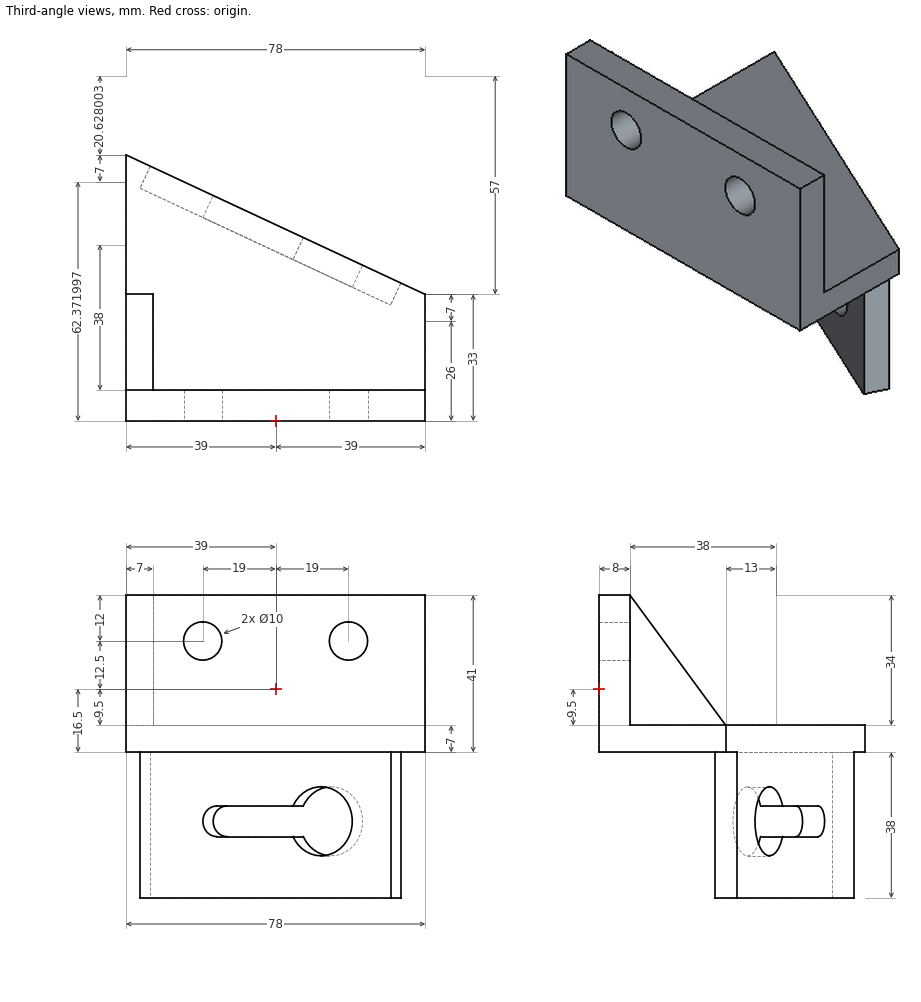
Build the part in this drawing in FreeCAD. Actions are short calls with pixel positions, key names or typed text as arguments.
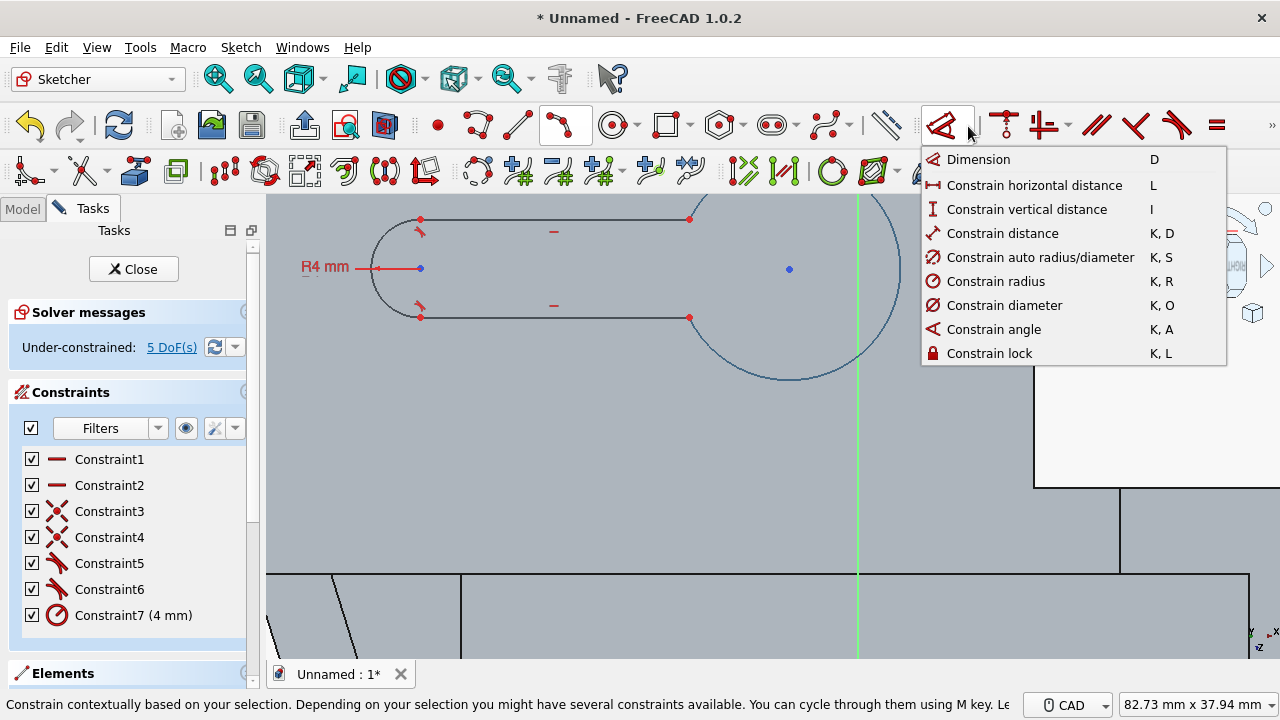
click(1074, 281)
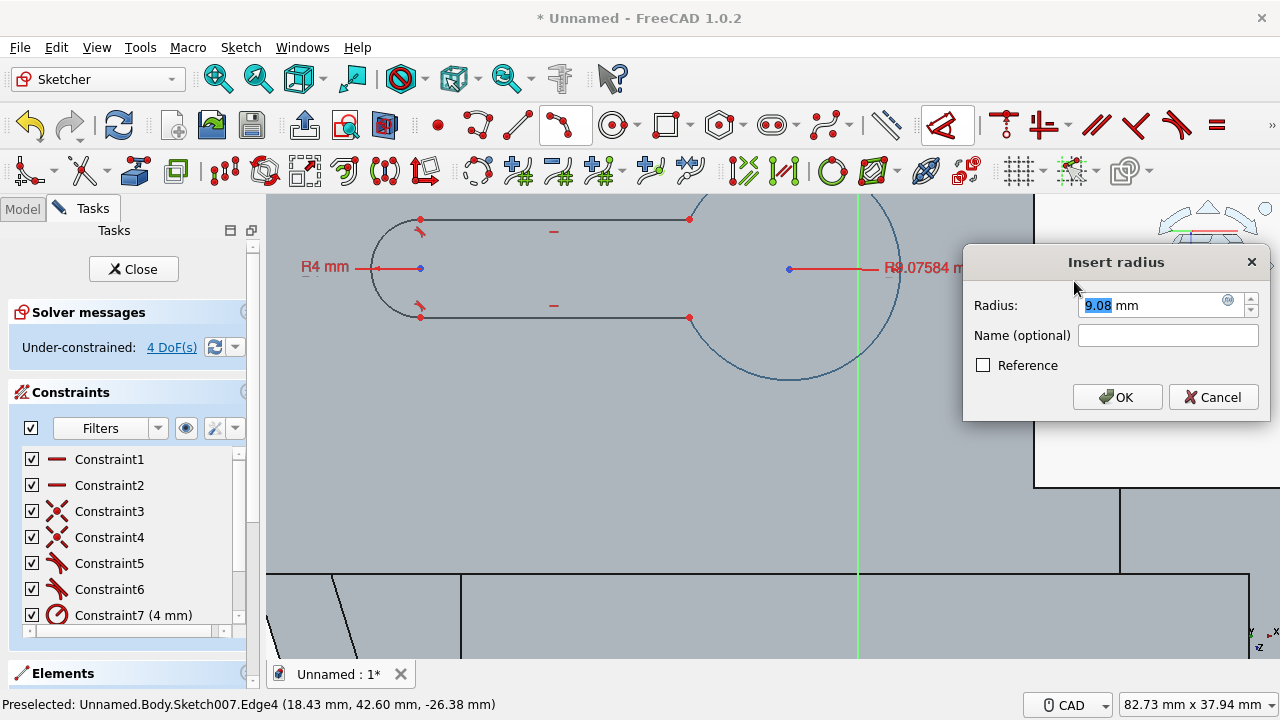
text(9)
key(Return)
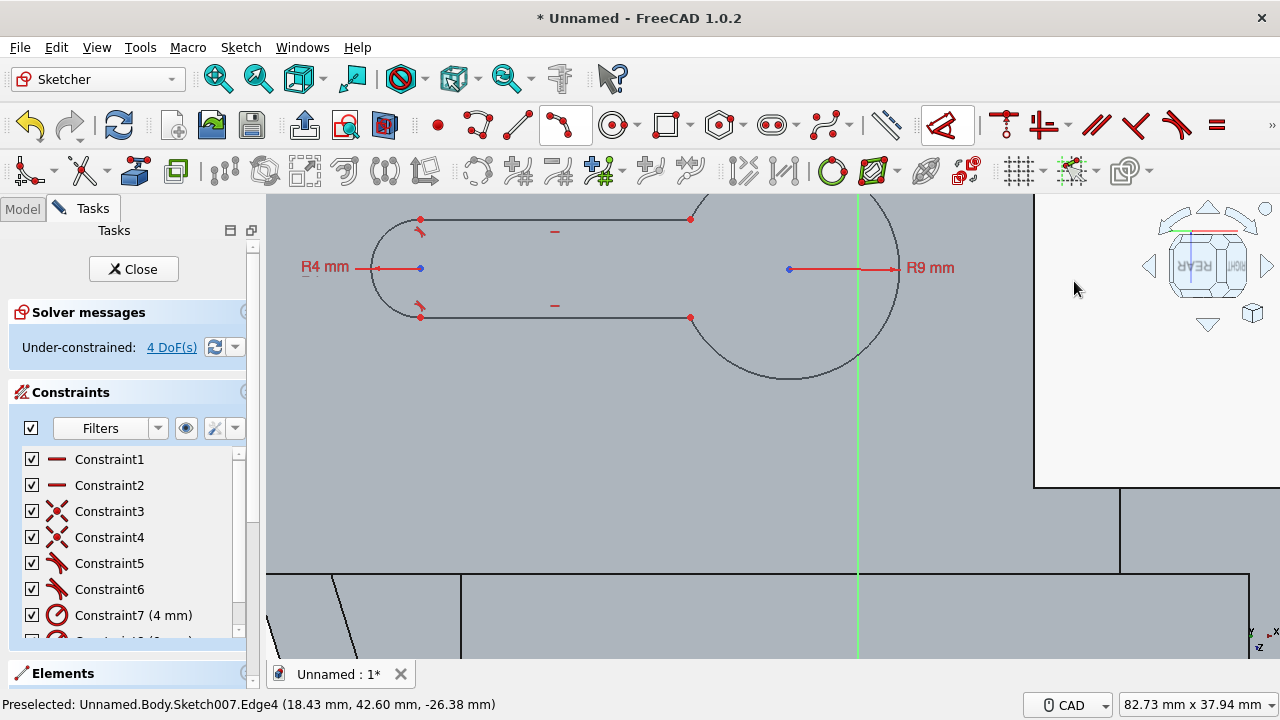
scroll(844, 369, down, 2)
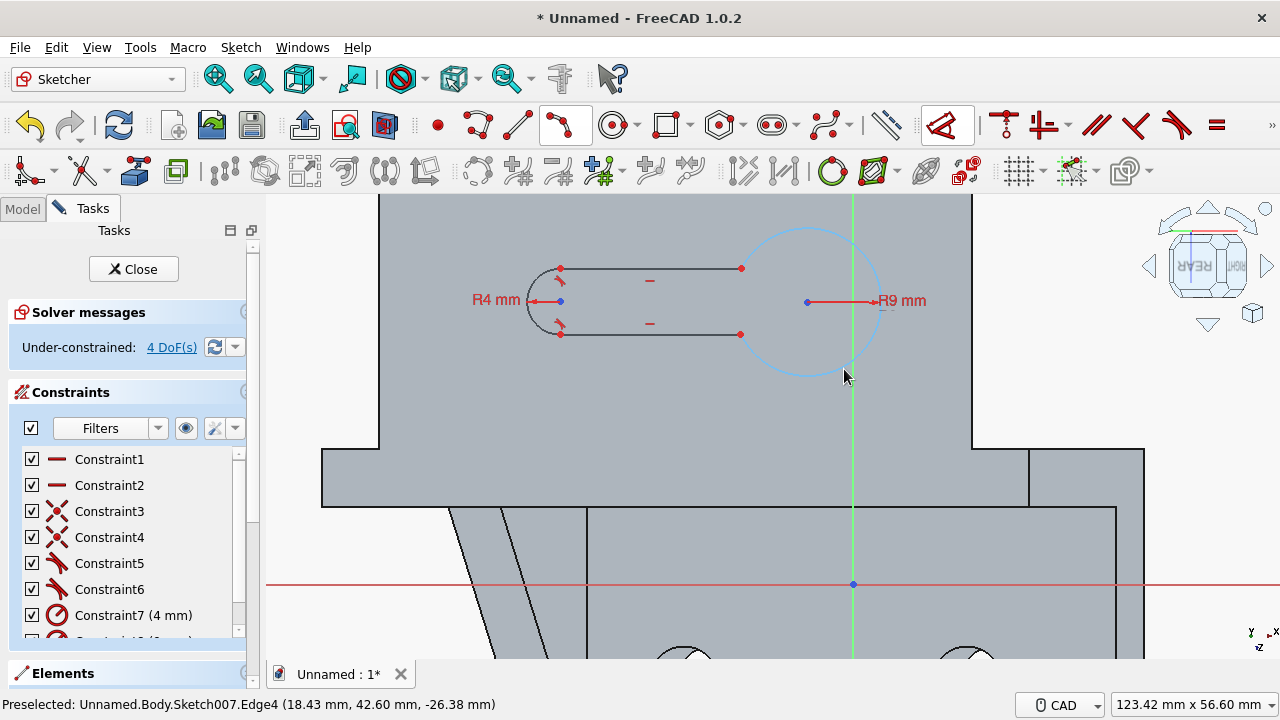
click(741, 269)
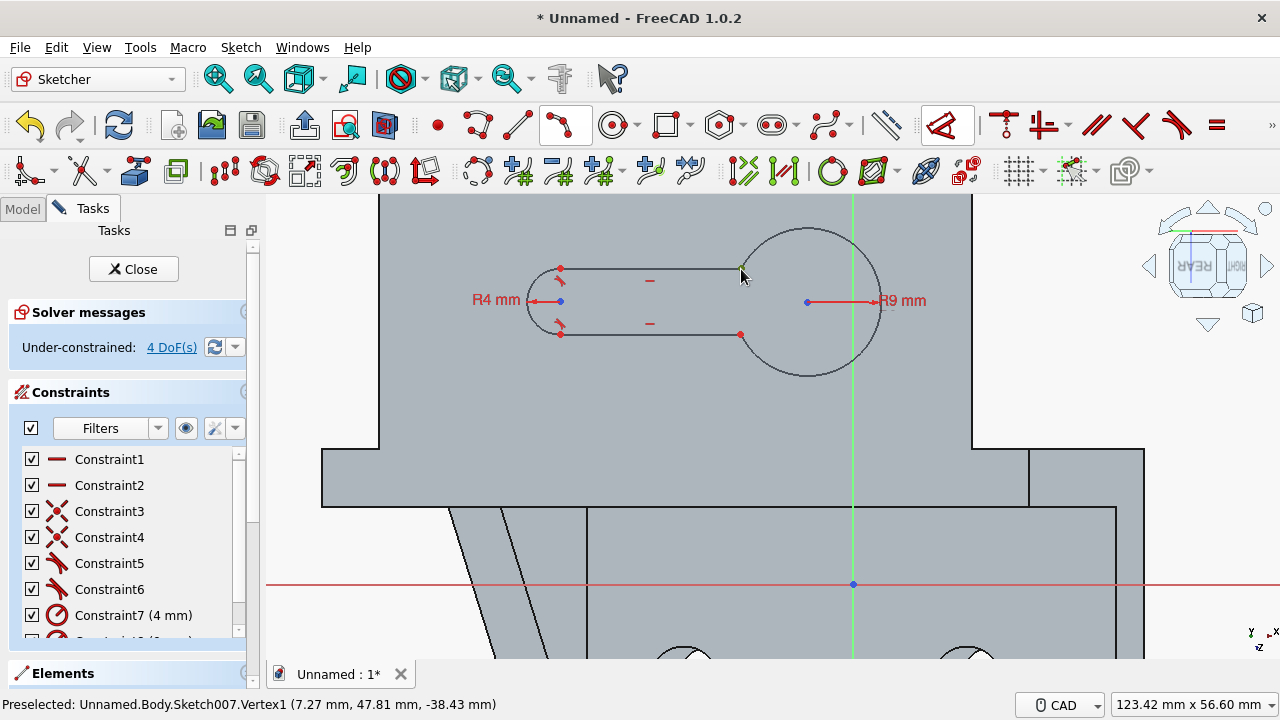
key(i)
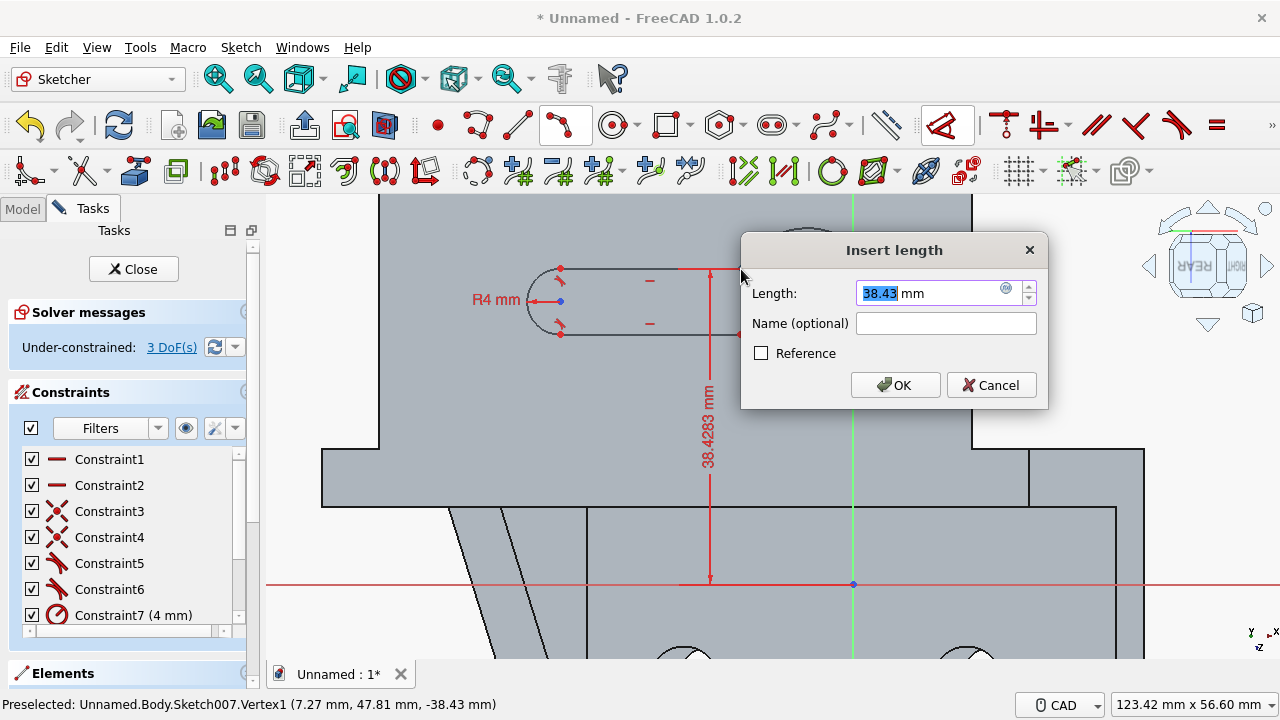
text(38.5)
key(Return)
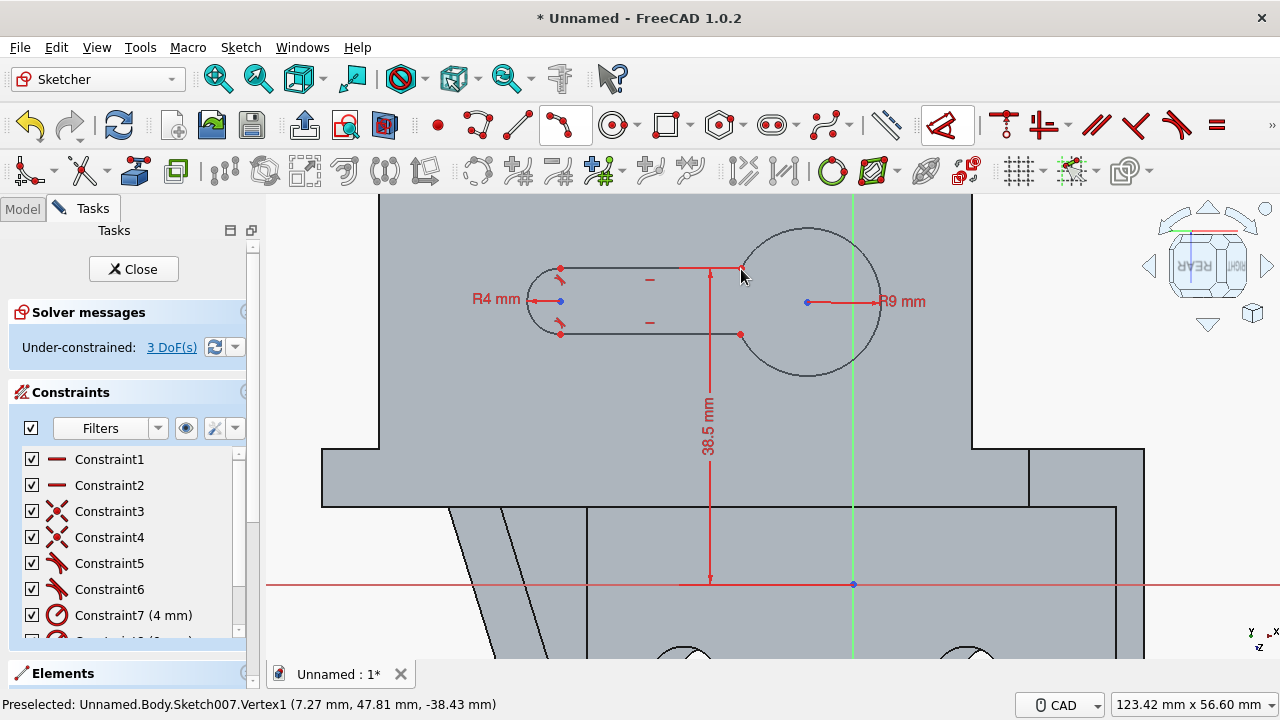
click(807, 302)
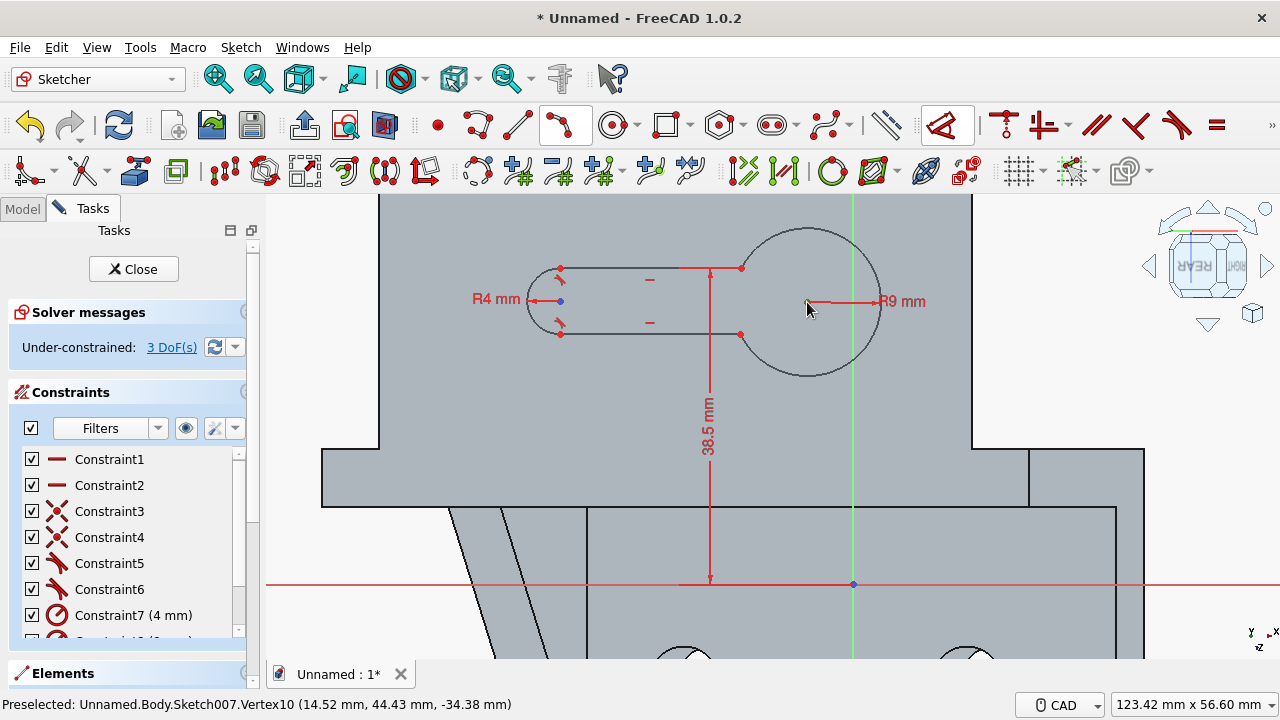
click(968, 126)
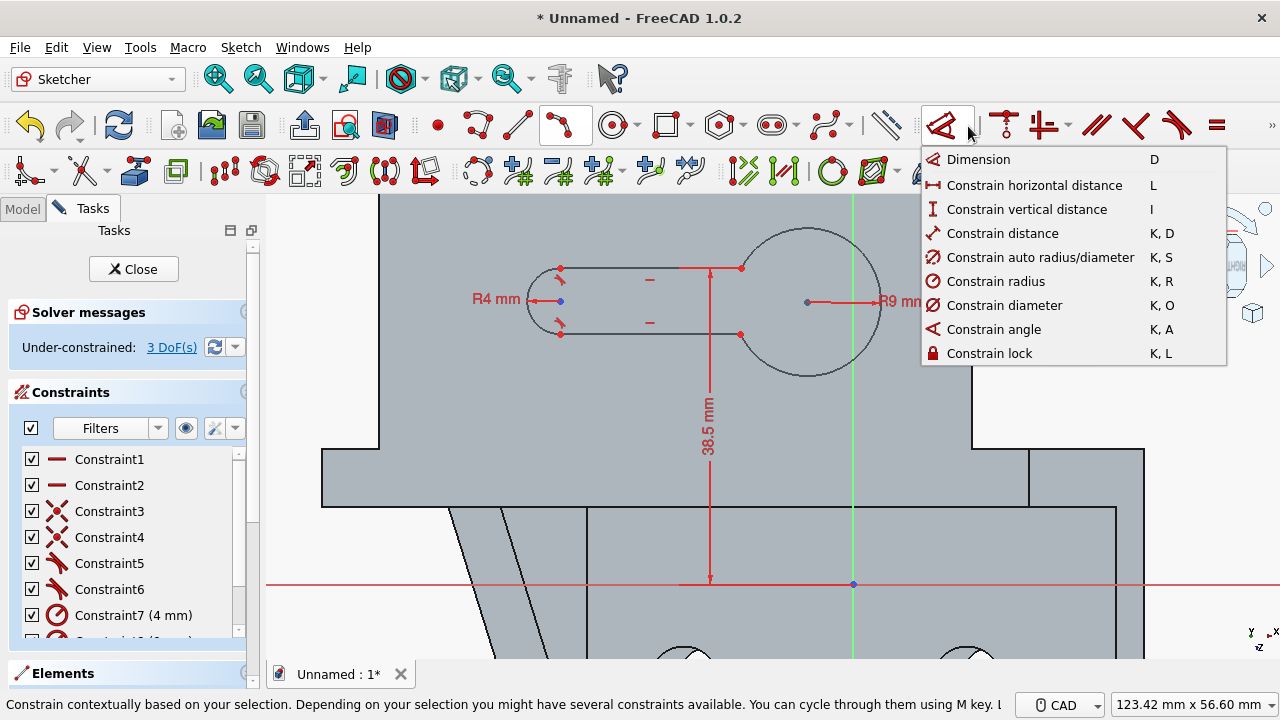
click(1074, 209)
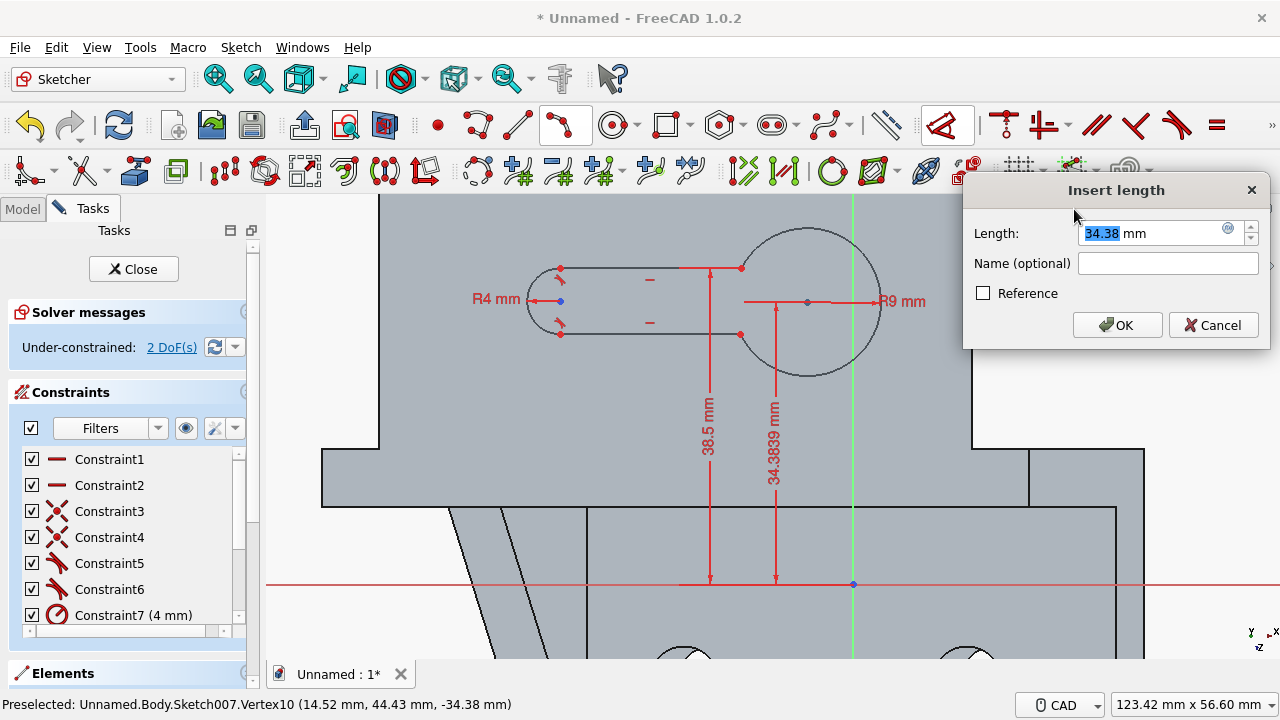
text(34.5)
key(Return)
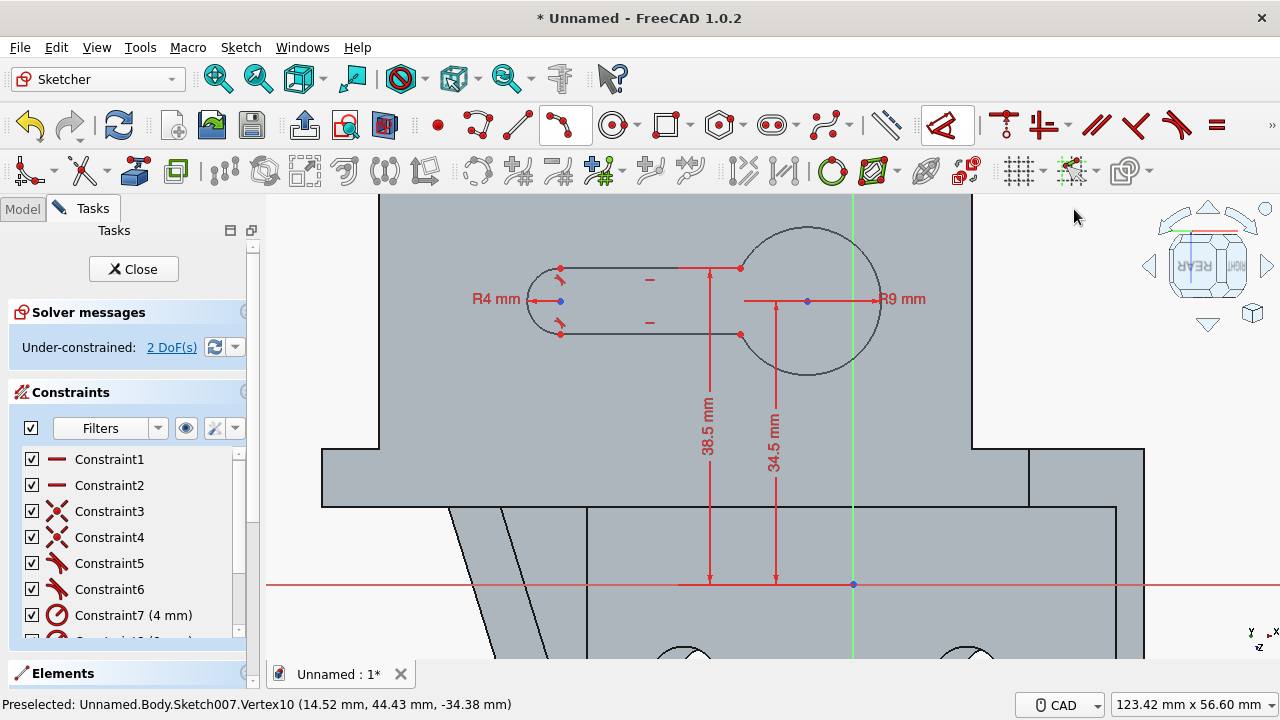
click(687, 268)